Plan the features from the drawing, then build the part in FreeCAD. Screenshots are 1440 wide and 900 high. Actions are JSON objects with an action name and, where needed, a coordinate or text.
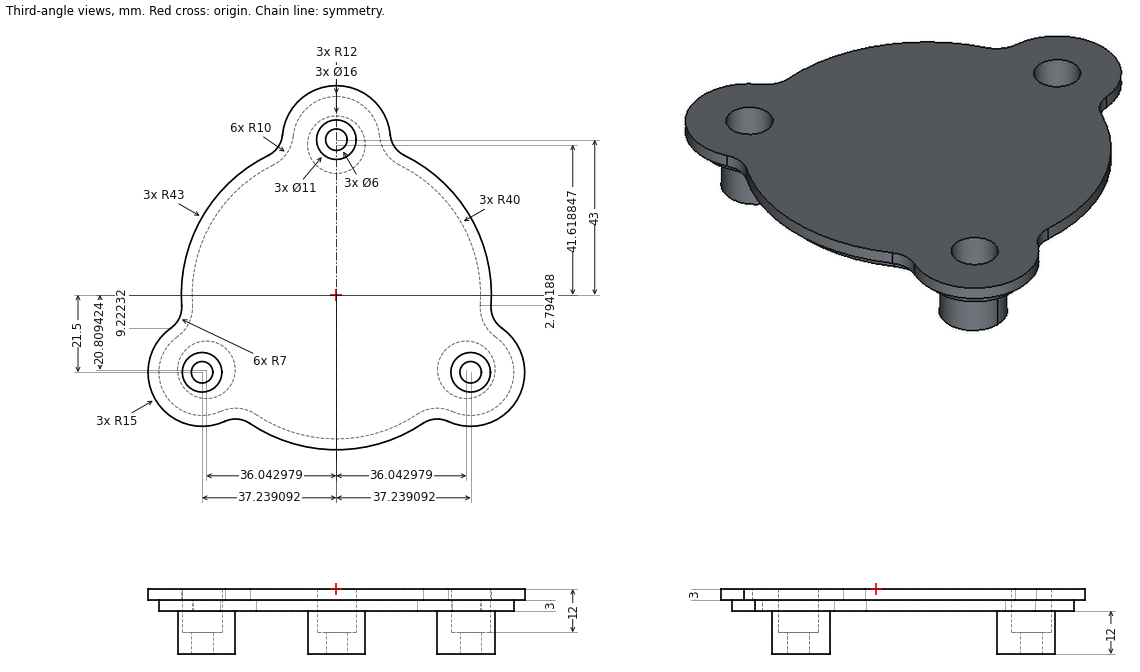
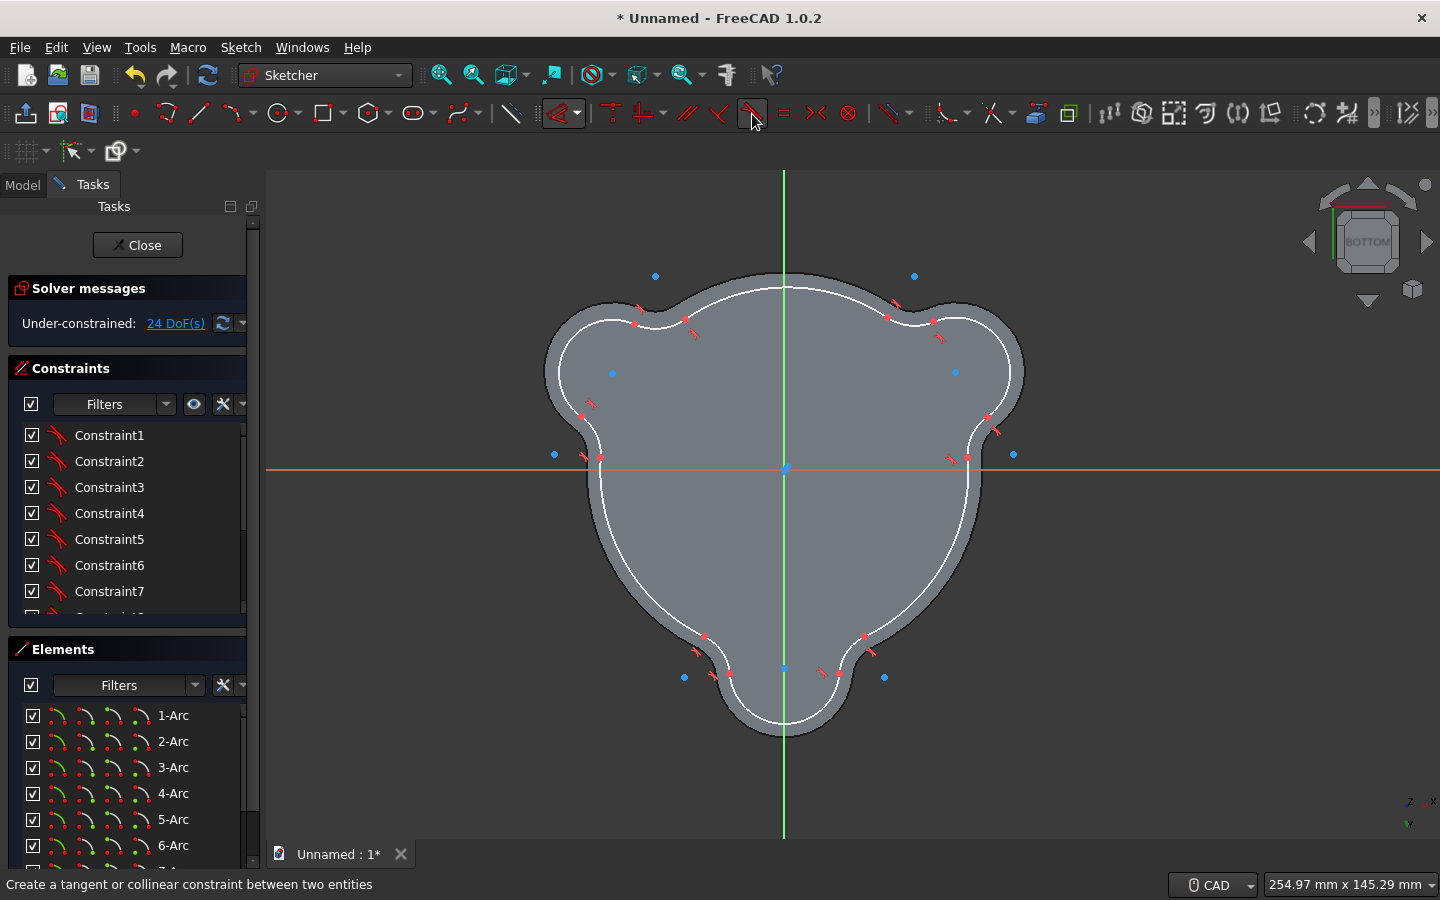
{"action": "left_click", "coordinate": [917, 598]}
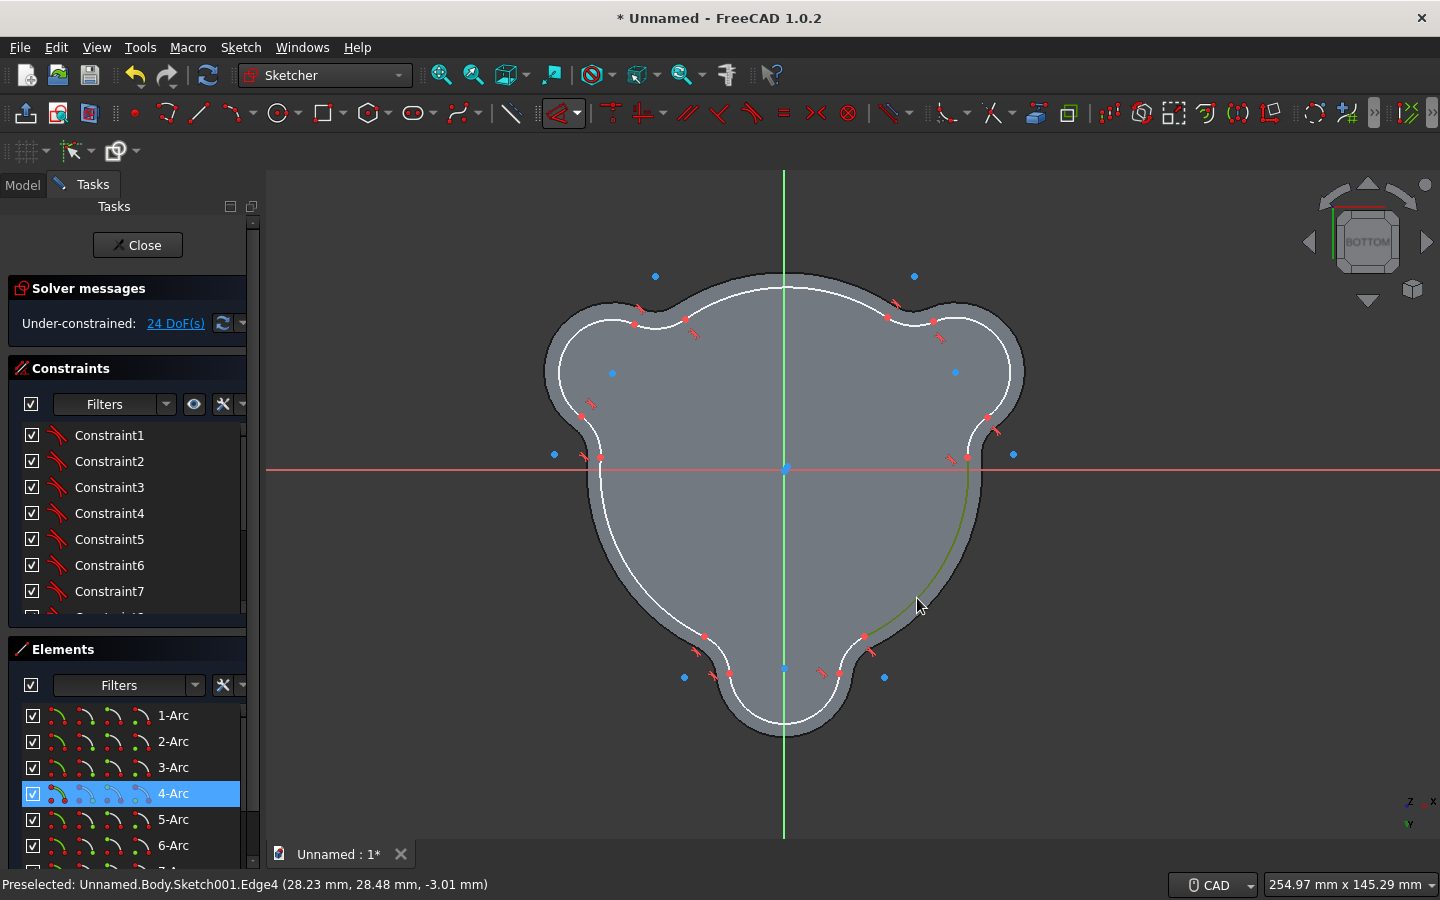
{"action": "left_click", "coordinate": [828, 292]}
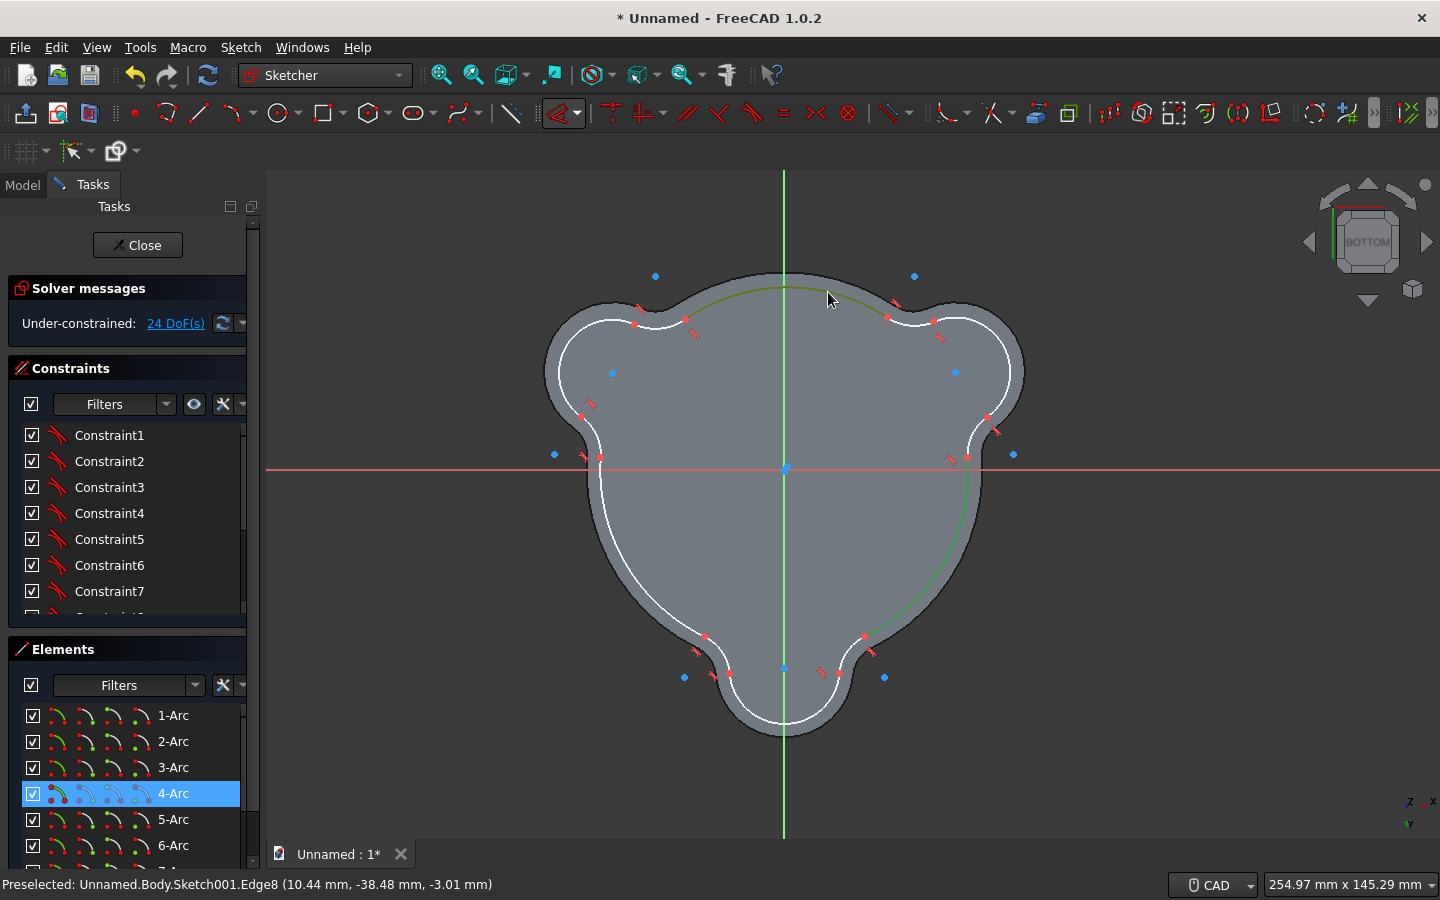
{"action": "left_click", "coordinate": [612, 114]}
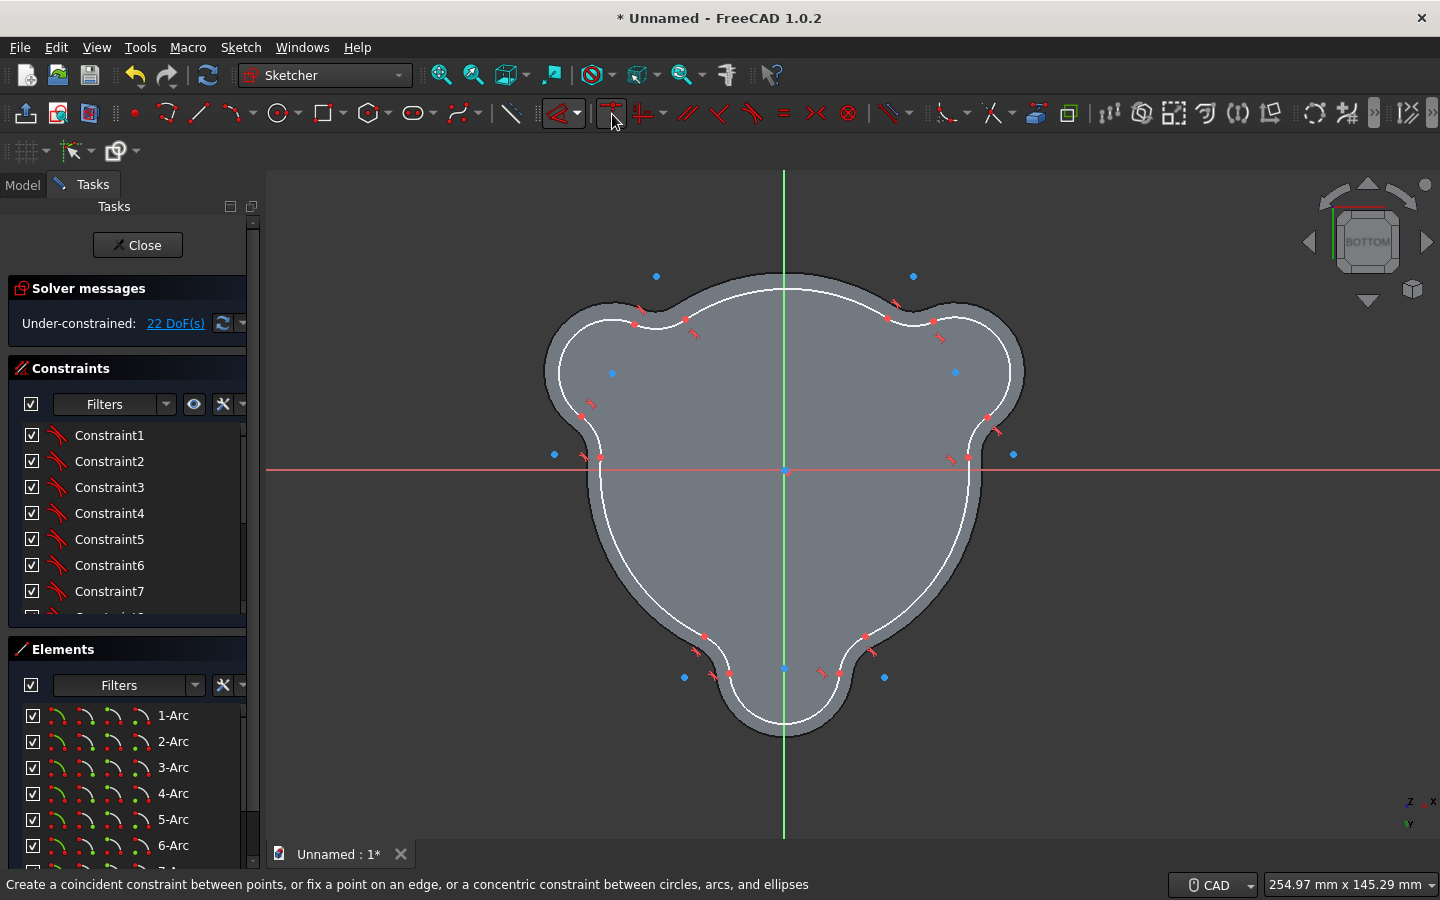
{"action": "left_click", "coordinate": [918, 599]}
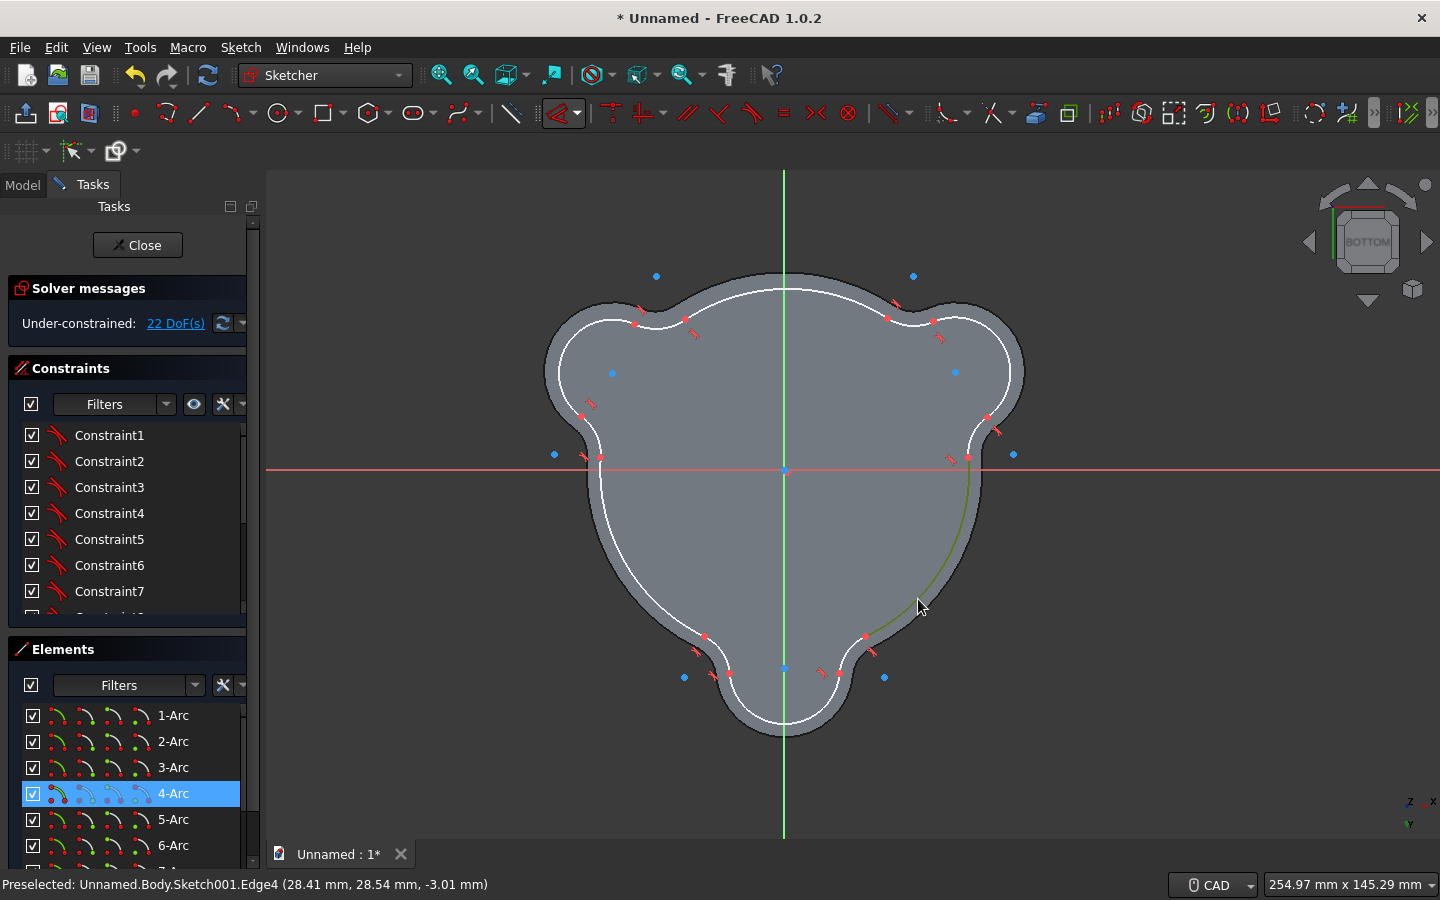
{"action": "left_click", "coordinate": [608, 523]}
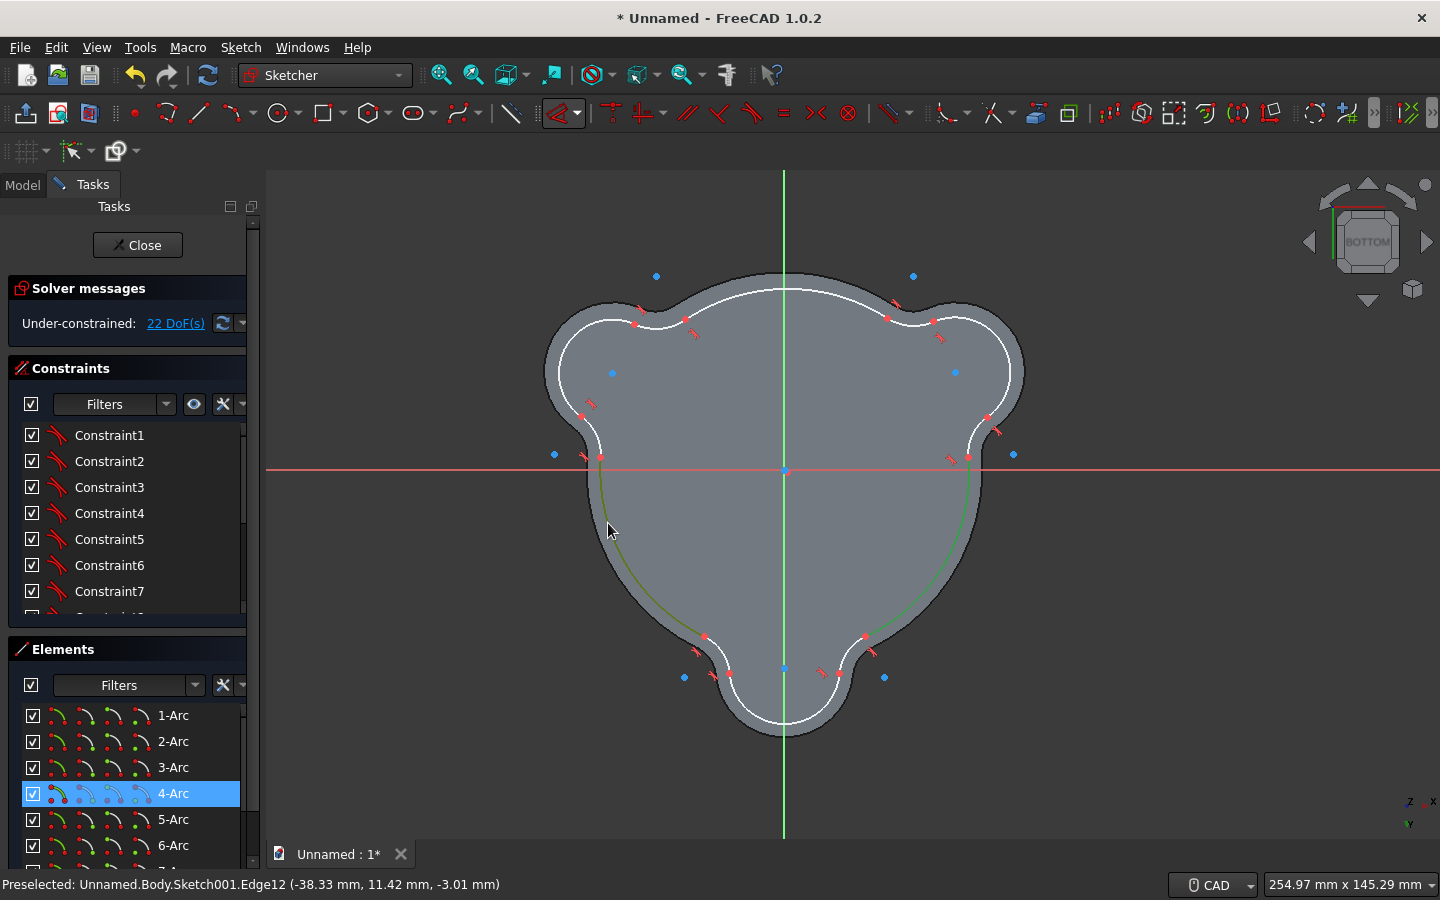
{"action": "left_click", "coordinate": [612, 114]}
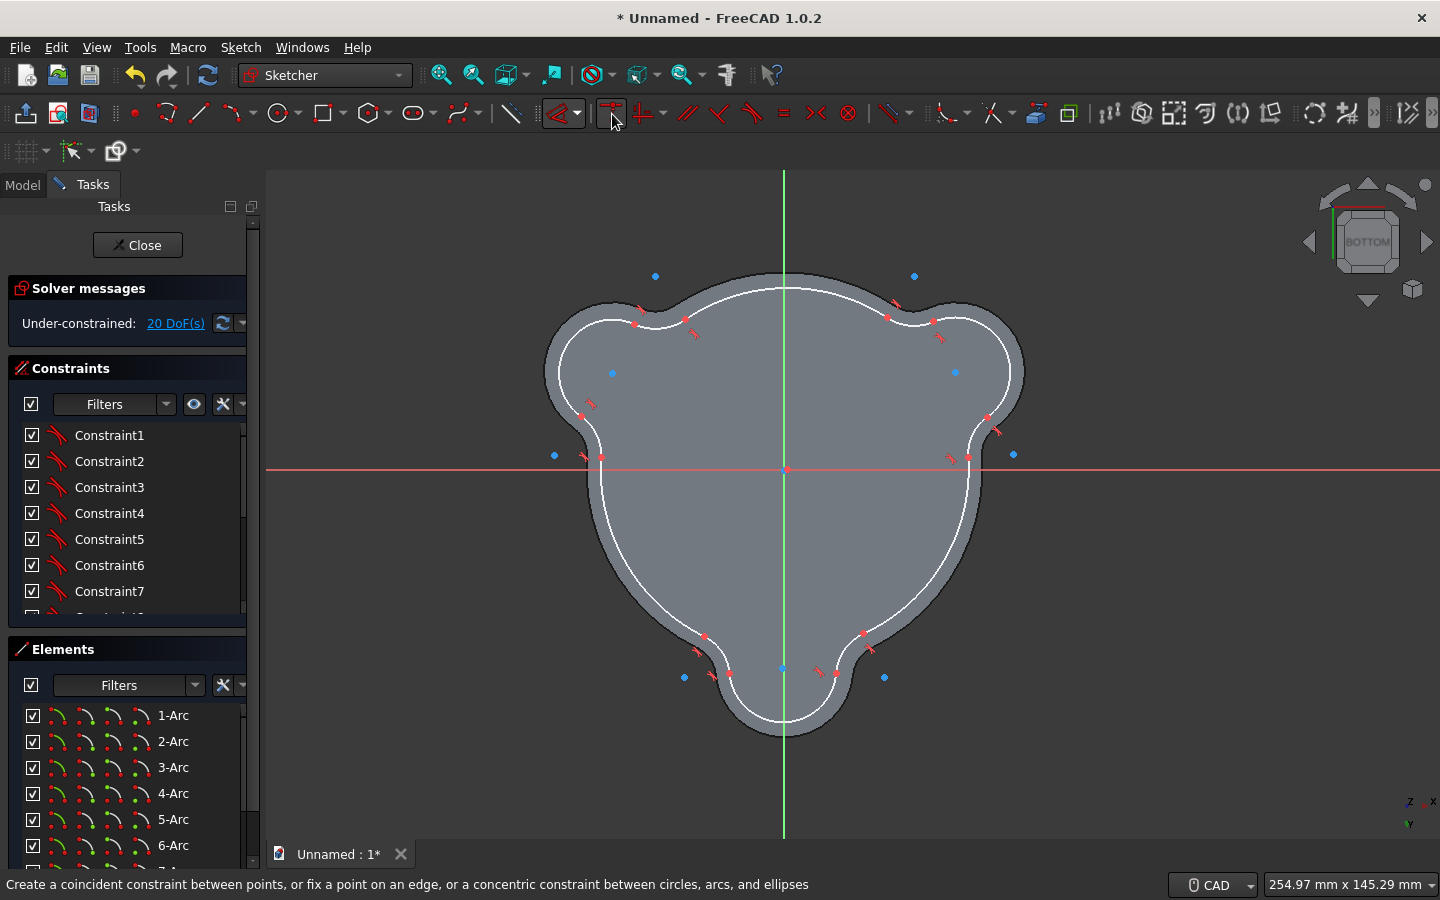
{"action": "left_click_drag", "start_coordinate": [774, 459], "coordinate": [798, 480]}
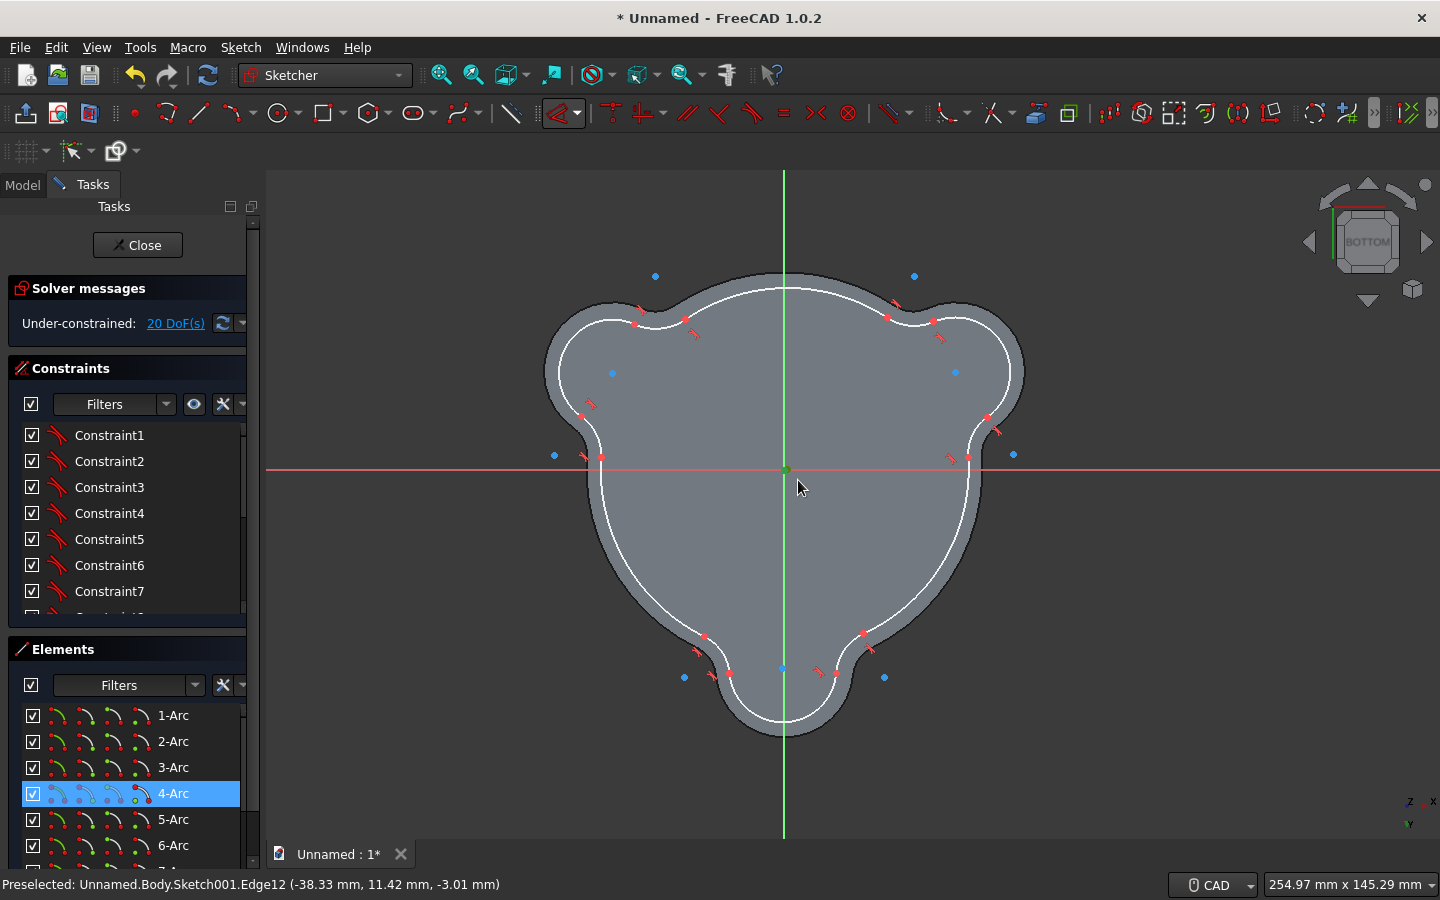
{"action": "left_click", "coordinate": [612, 114]}